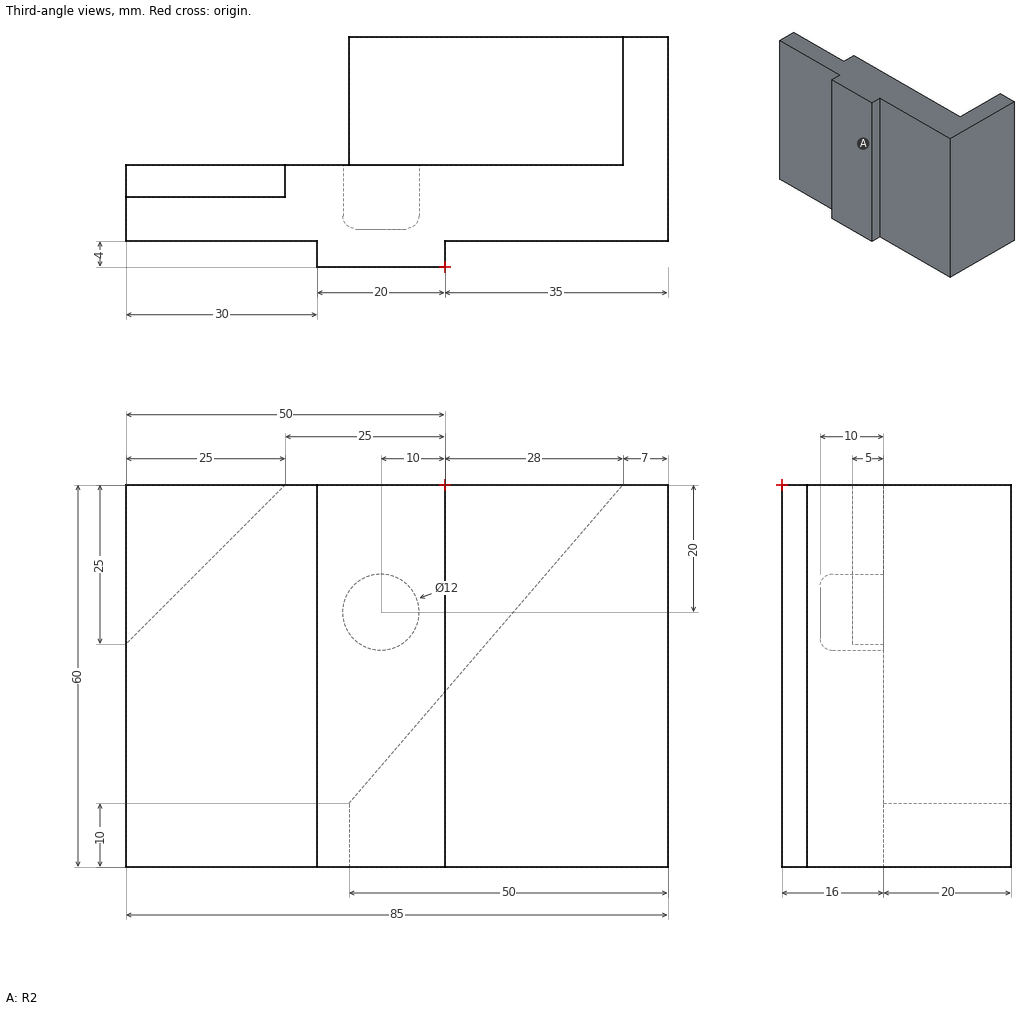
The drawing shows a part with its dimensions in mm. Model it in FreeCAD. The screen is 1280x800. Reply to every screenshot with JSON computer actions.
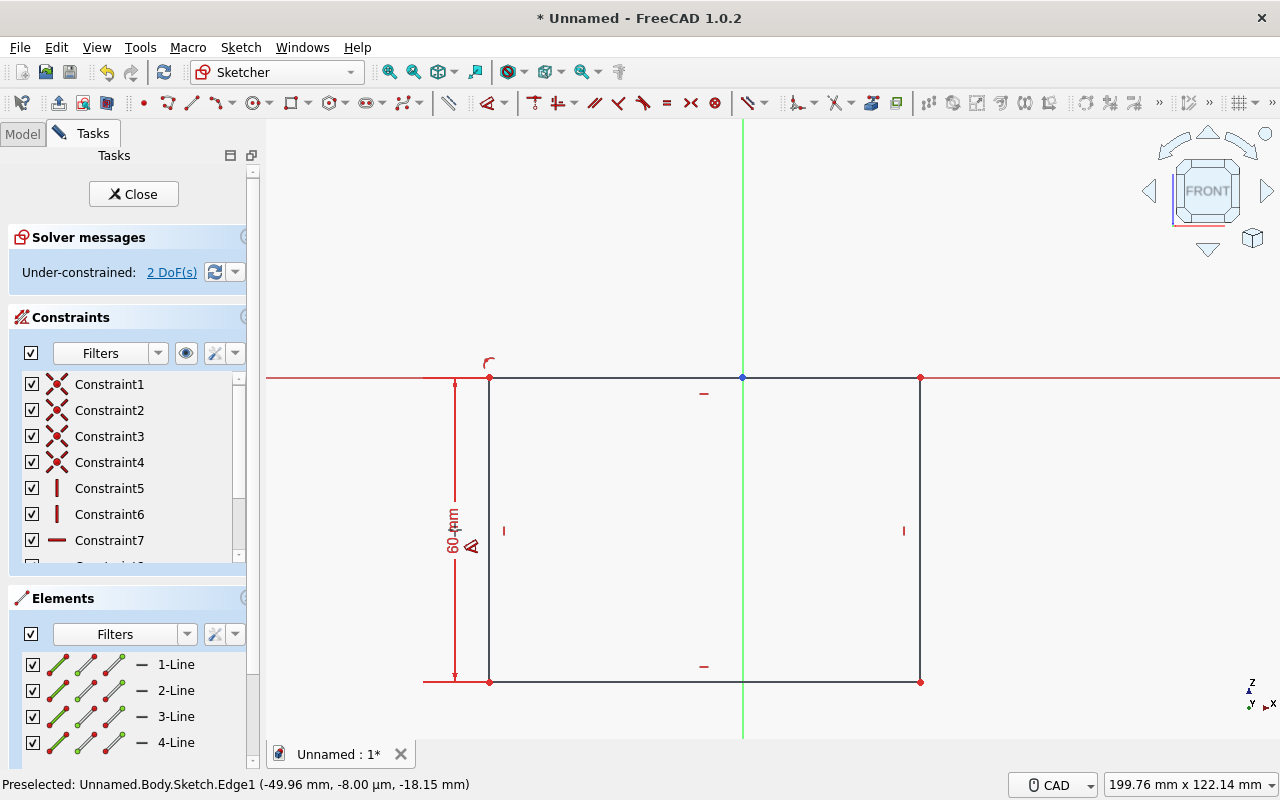
{"action": "left_click", "coordinate": [618, 682]}
{"action": "left_click", "coordinate": [705, 648]}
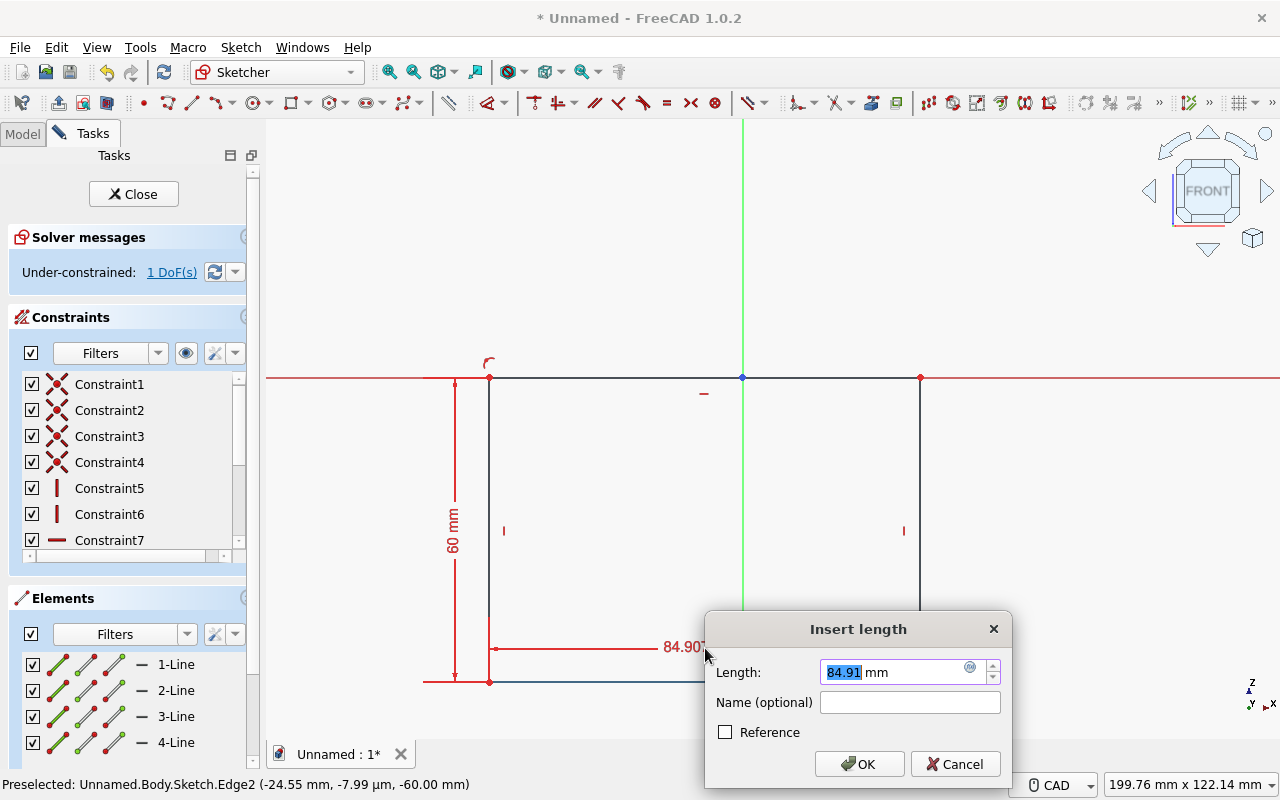
{"action": "type", "text": "85"}
{"action": "key", "text": "Return"}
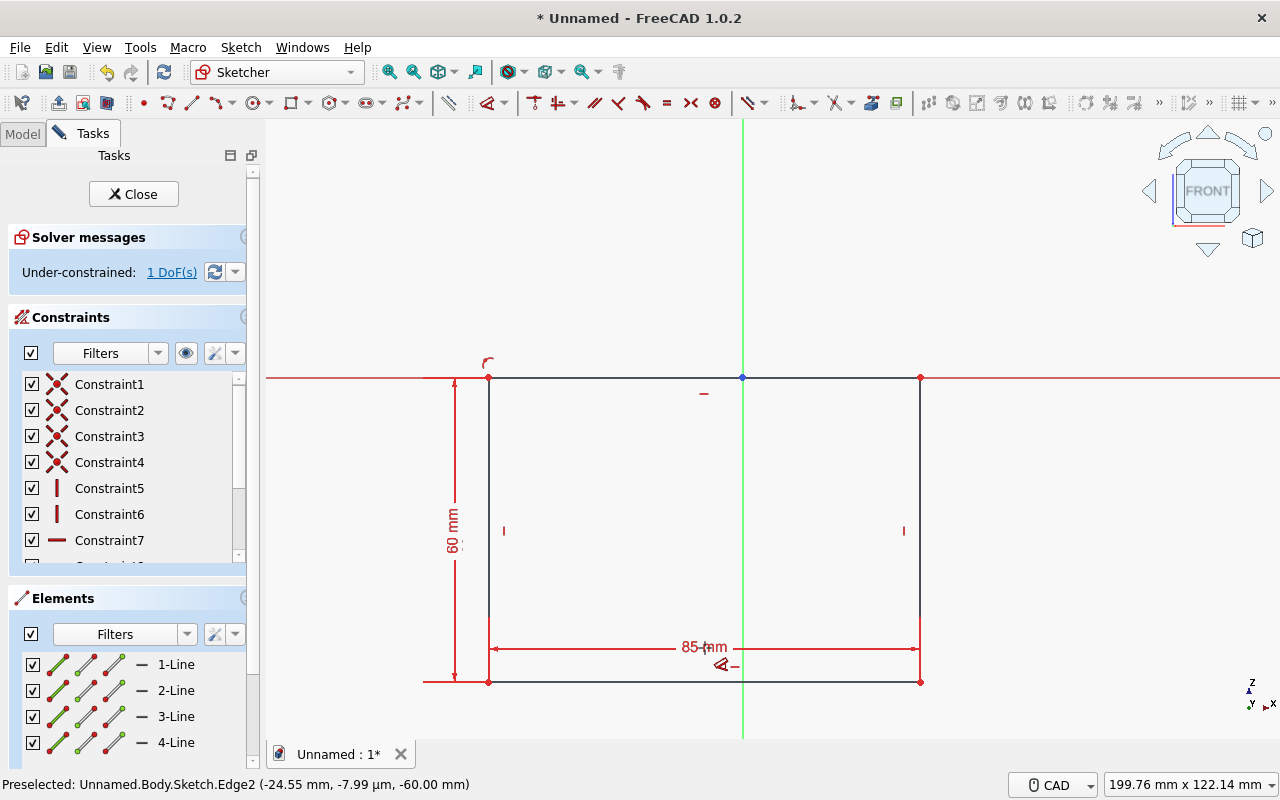
{"action": "left_click", "coordinate": [489, 378]}
{"action": "left_click", "coordinate": [616, 344]}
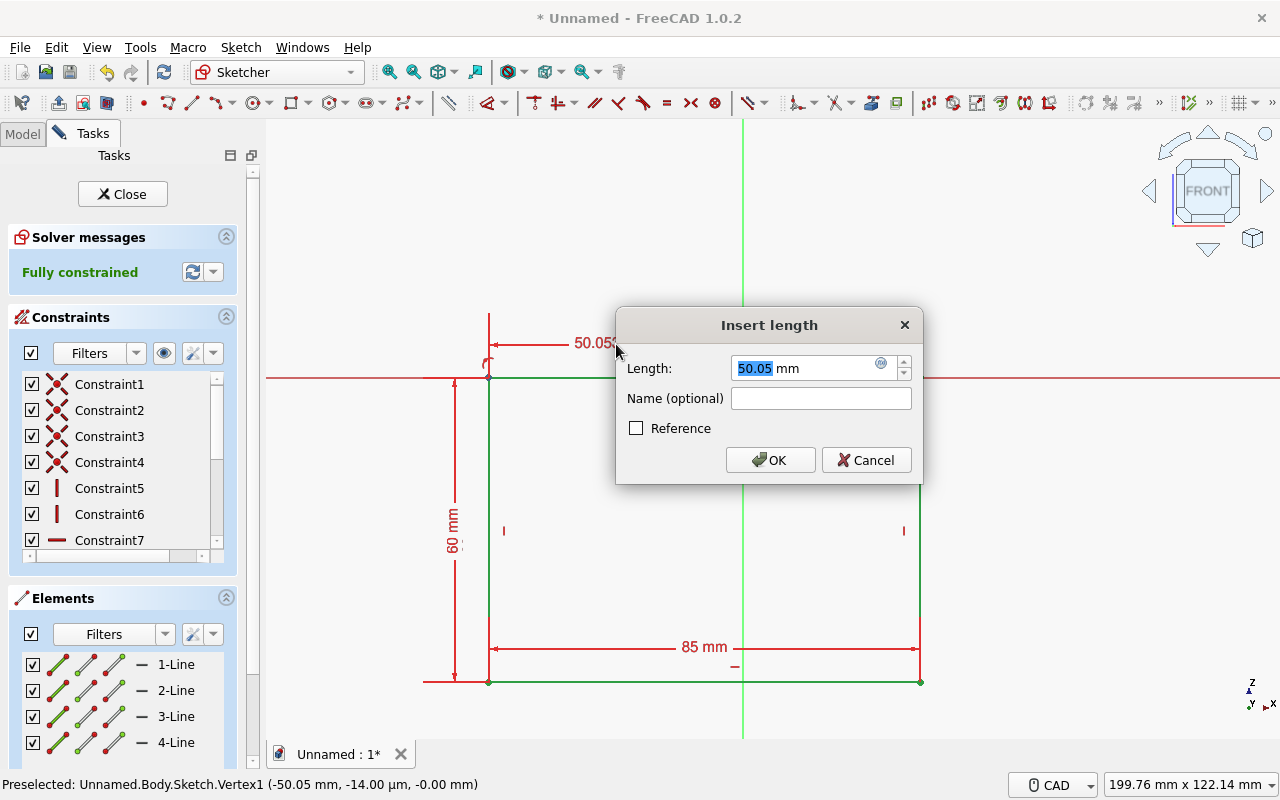
{"action": "type", "text": "50"}
{"action": "key", "text": "Return"}
{"action": "key", "text": "Escape"}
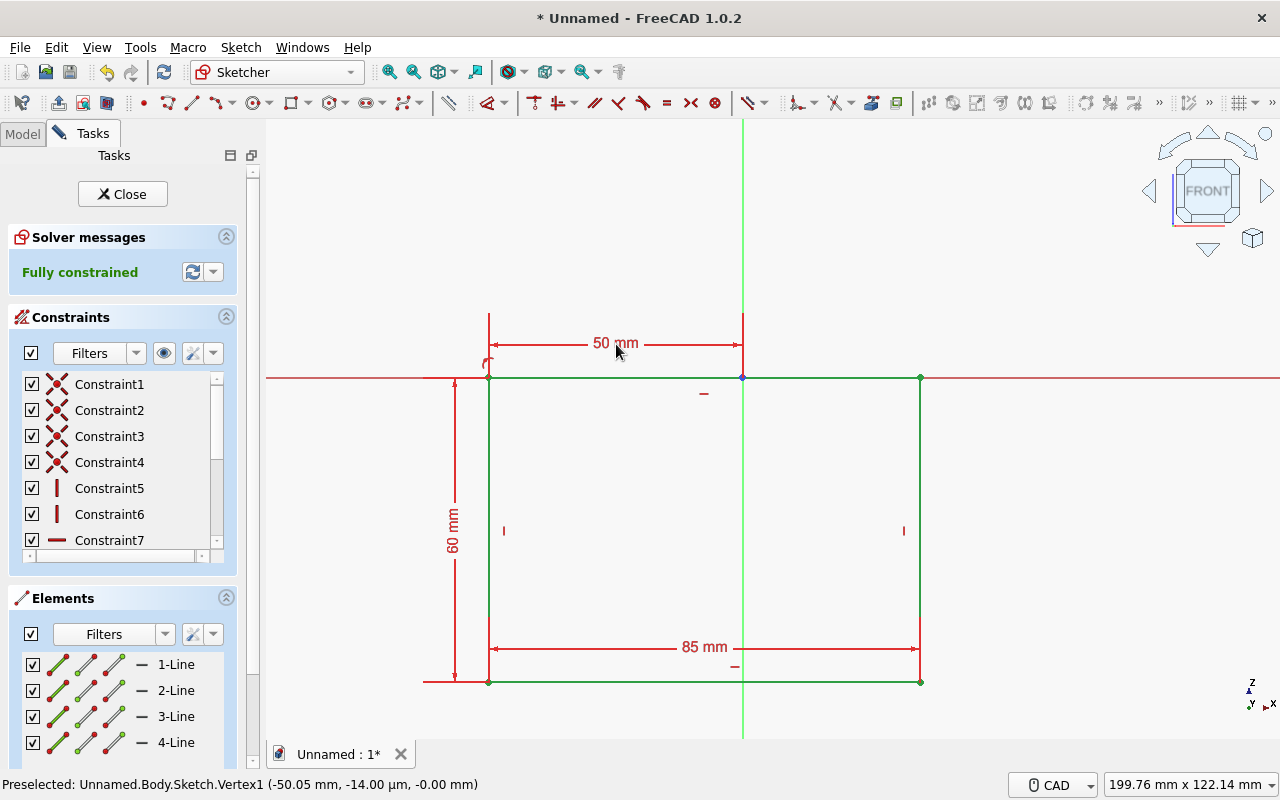
{"action": "left_click", "coordinate": [123, 194]}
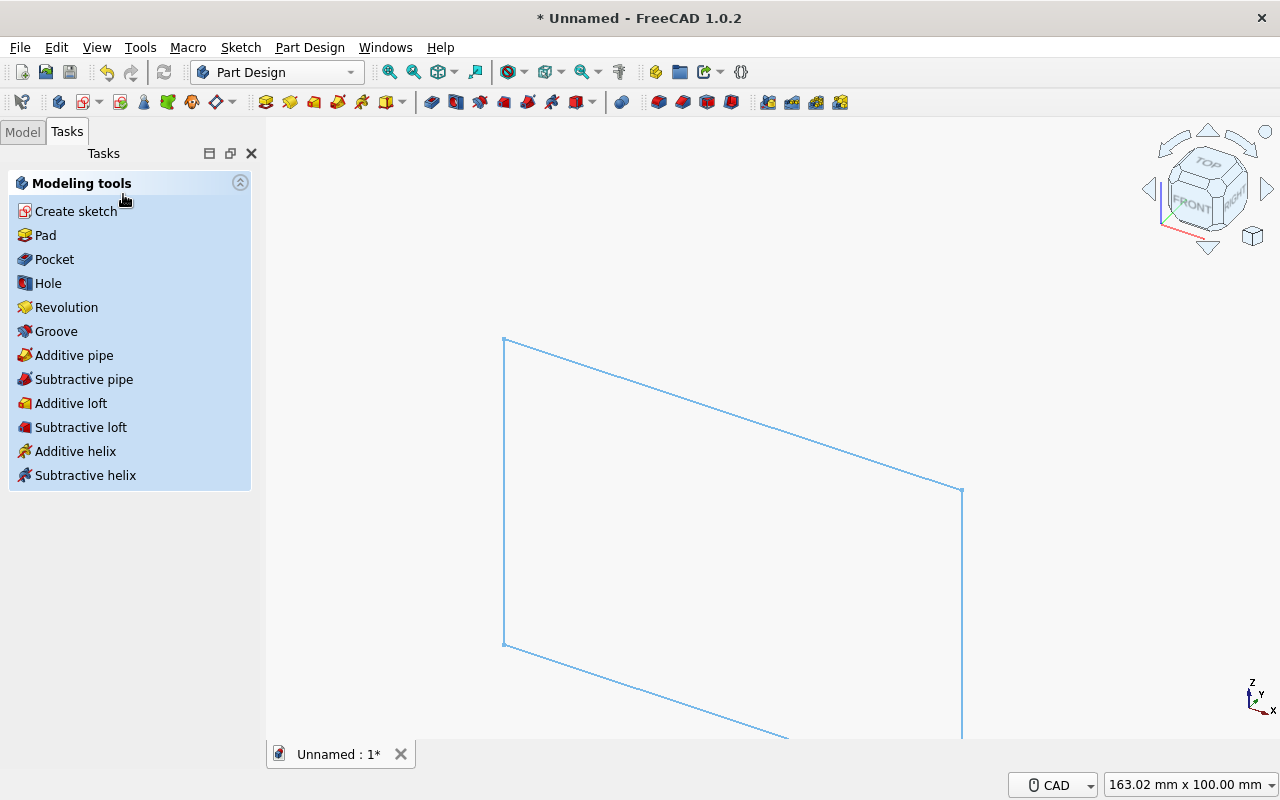
{"action": "left_click", "coordinate": [266, 102]}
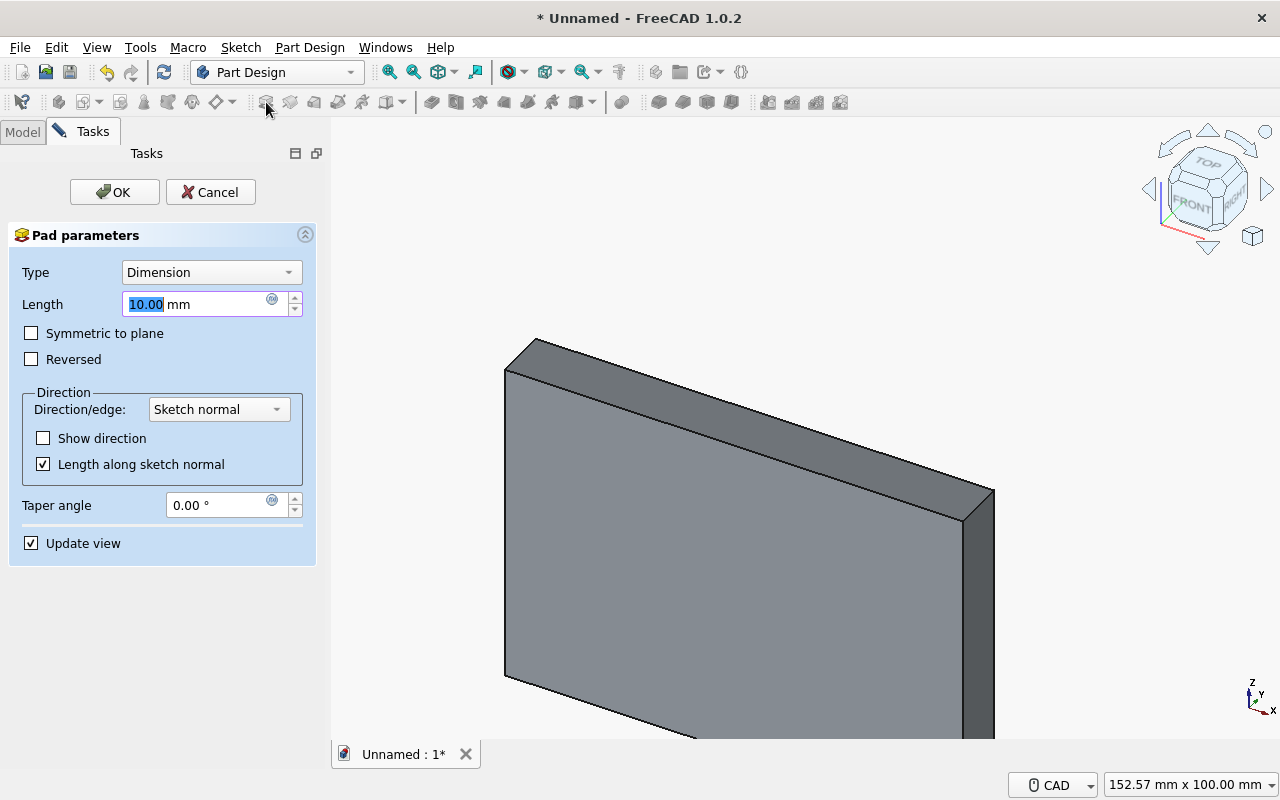
{"action": "type", "text": "16"}
{"action": "key", "text": "Tab"}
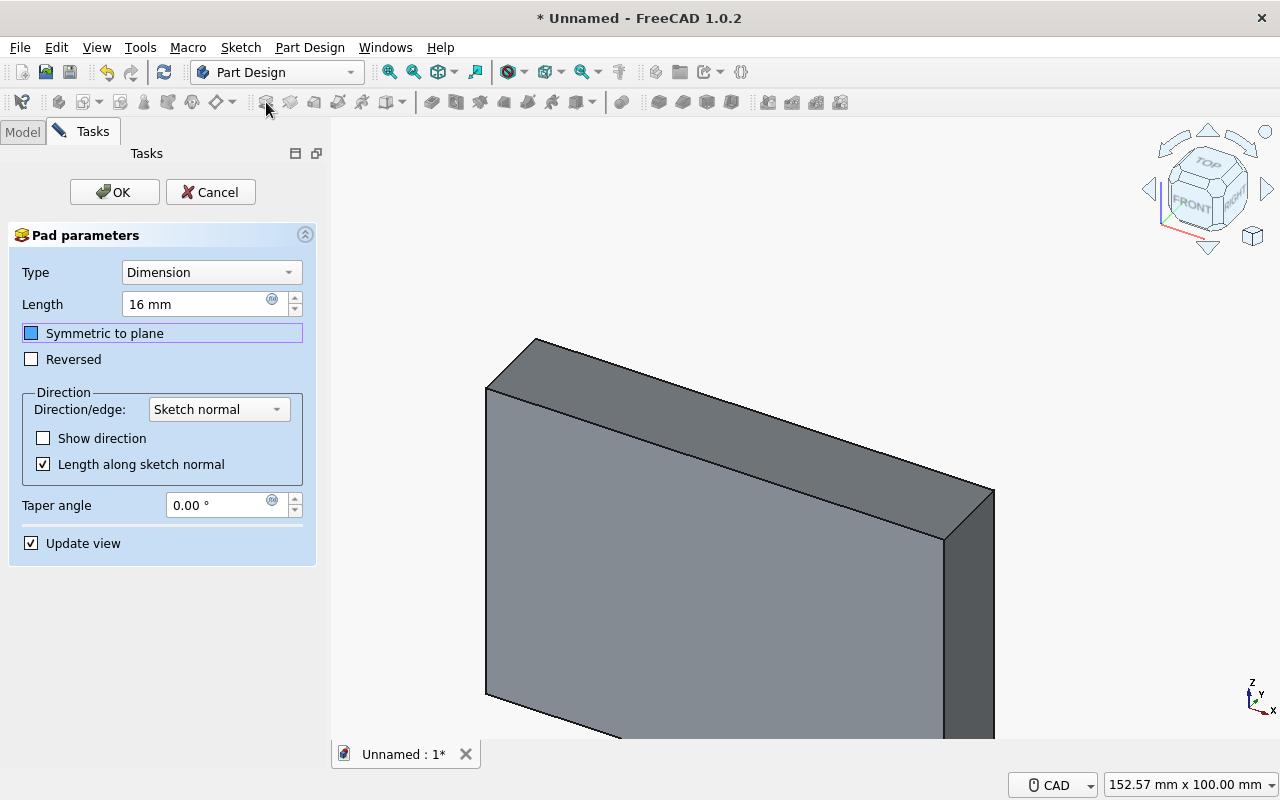
{"action": "left_click", "coordinate": [30, 359]}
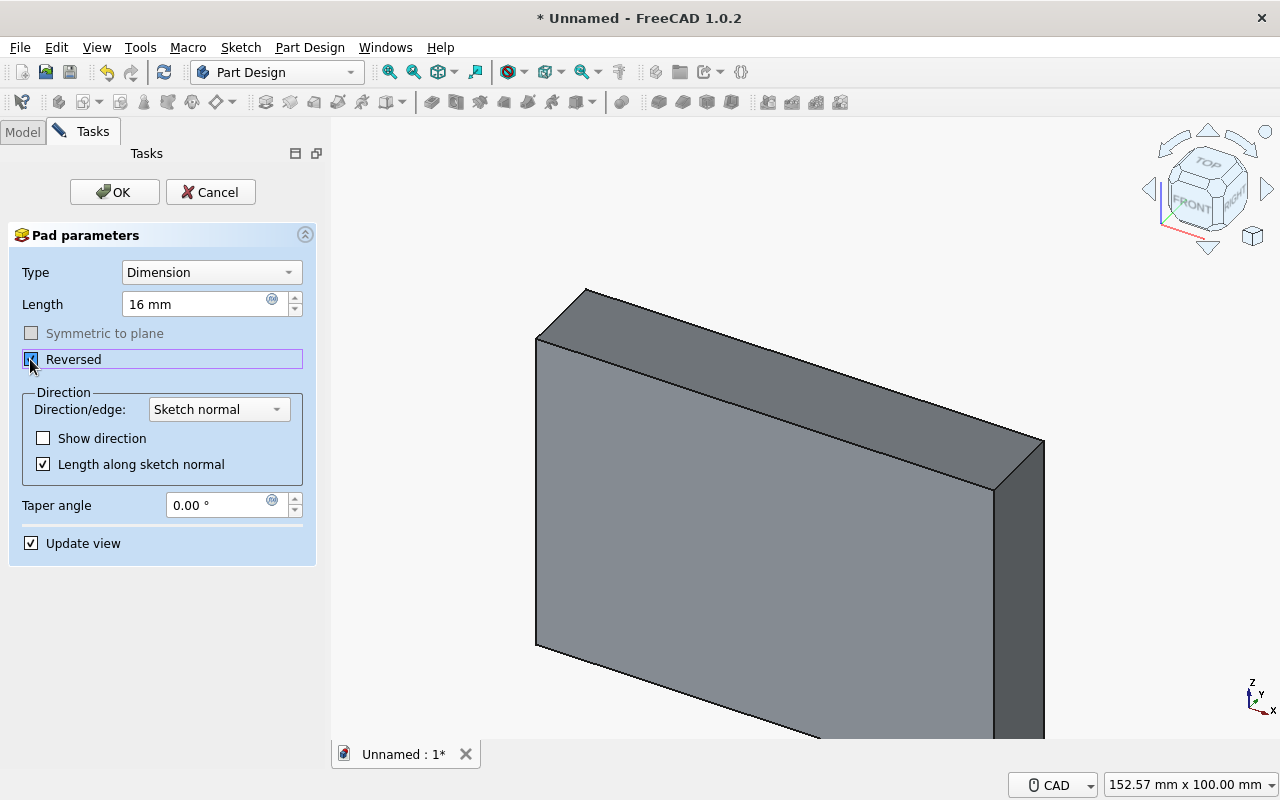
{"action": "left_click", "coordinate": [115, 192]}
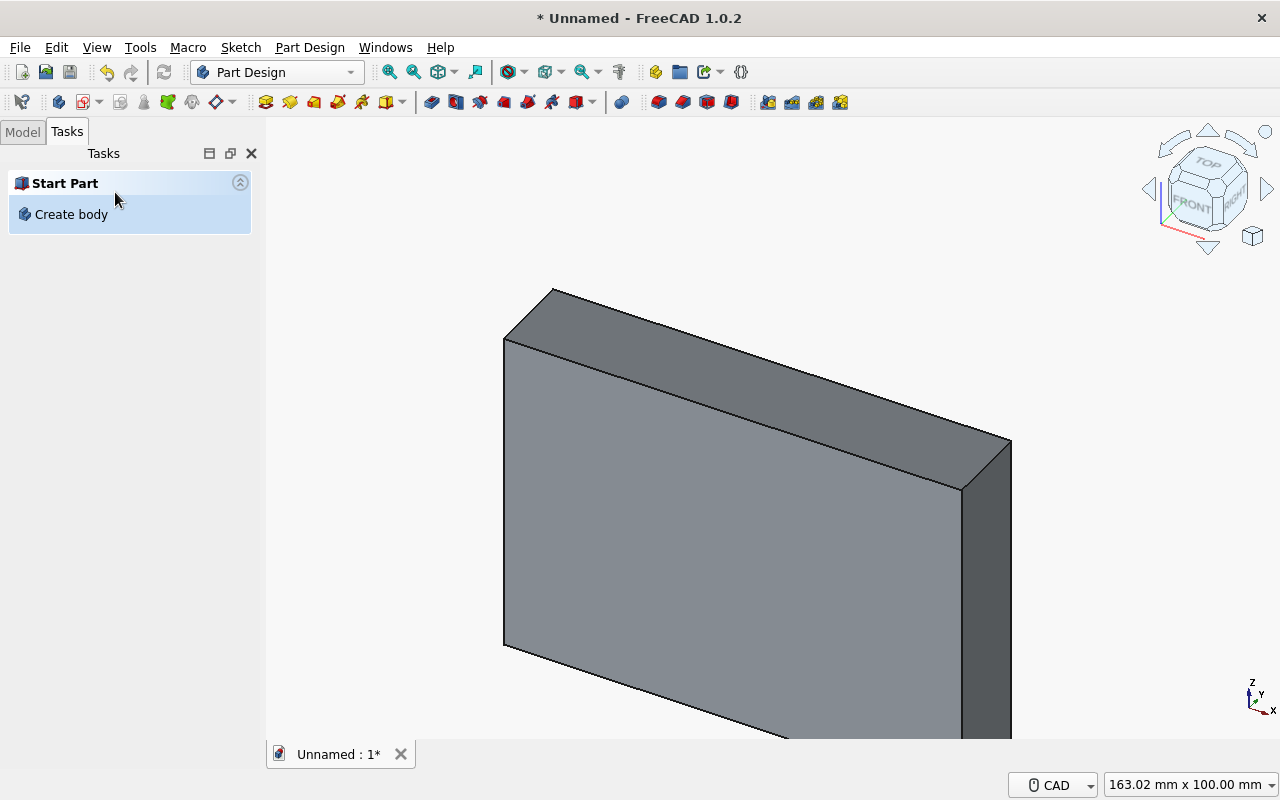
{"action": "left_click", "coordinate": [390, 72]}